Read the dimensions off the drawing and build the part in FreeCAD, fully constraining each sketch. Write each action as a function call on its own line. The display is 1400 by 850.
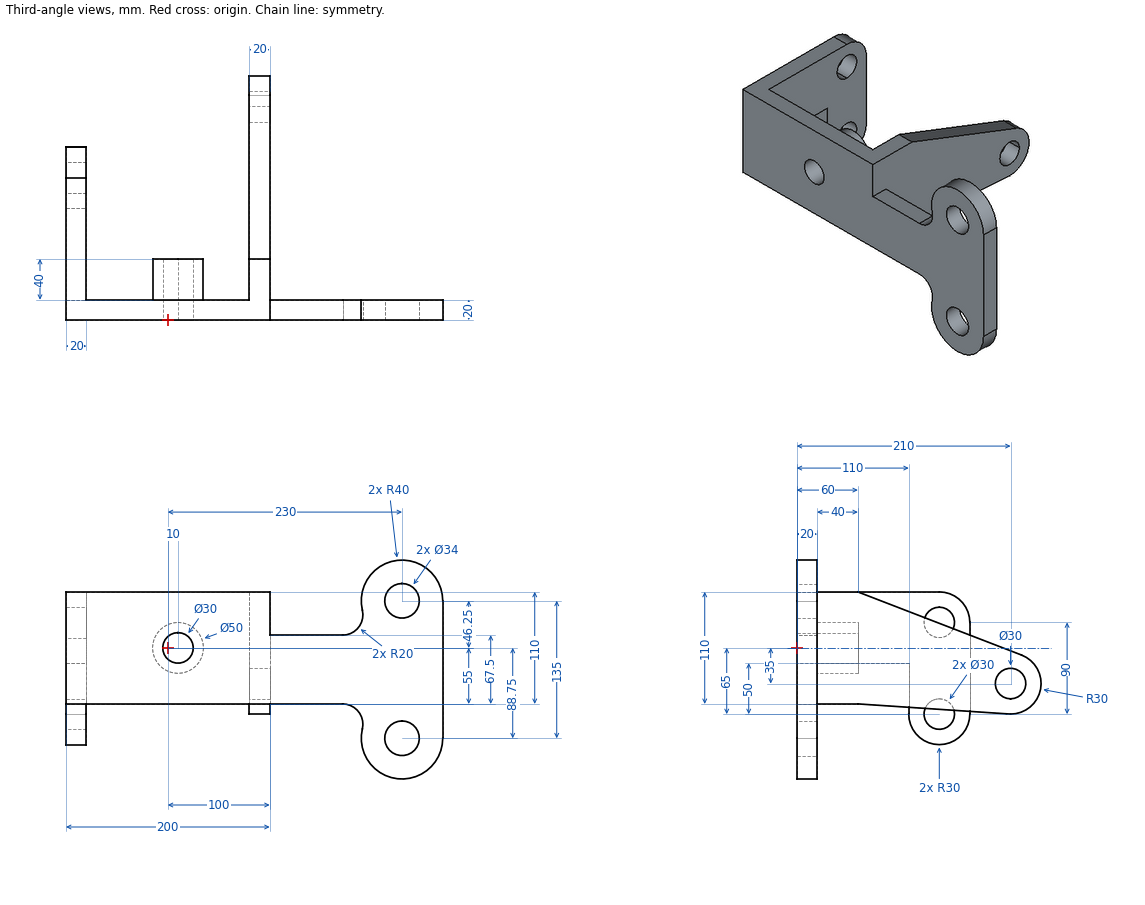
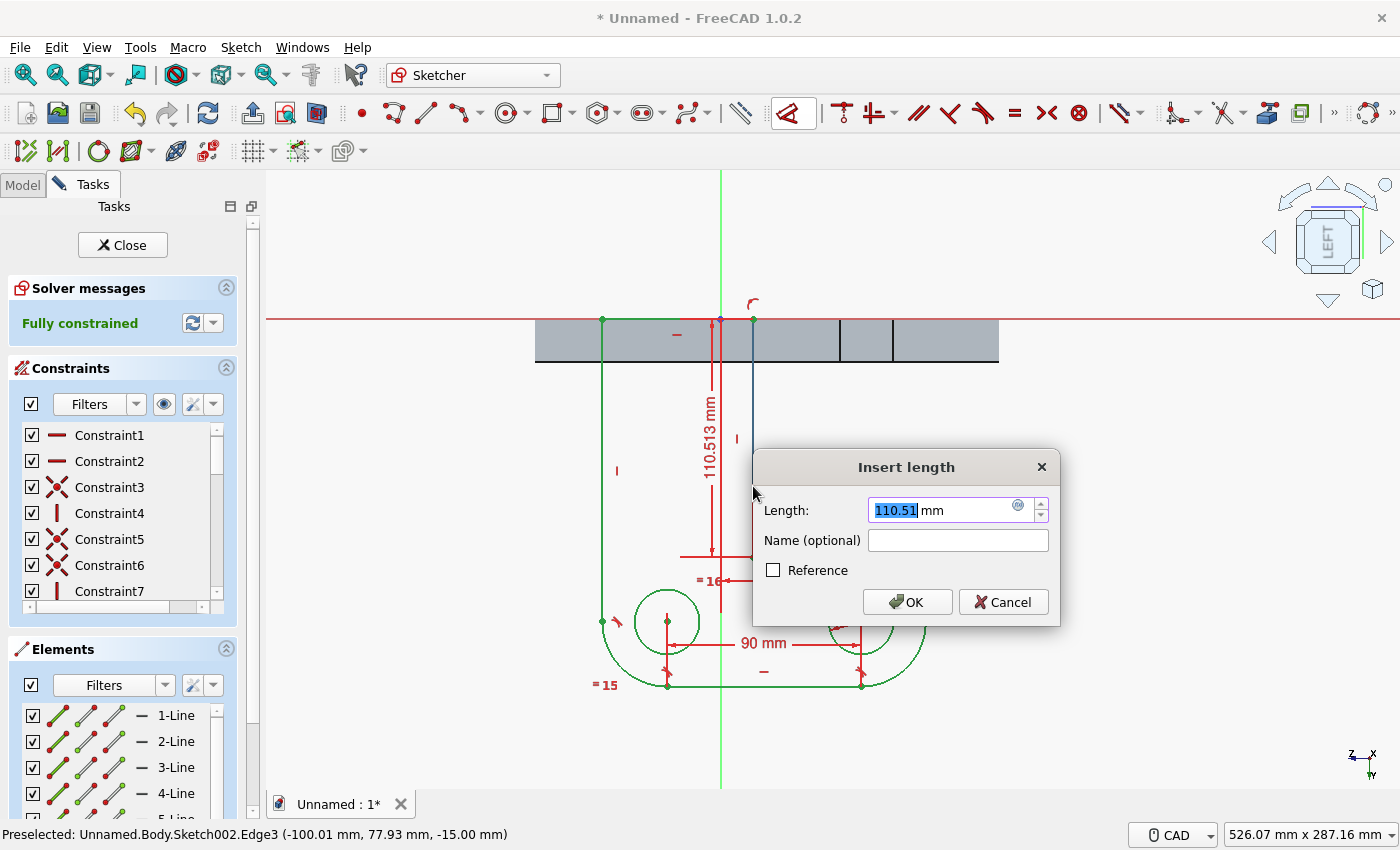
text(110)
key(Return)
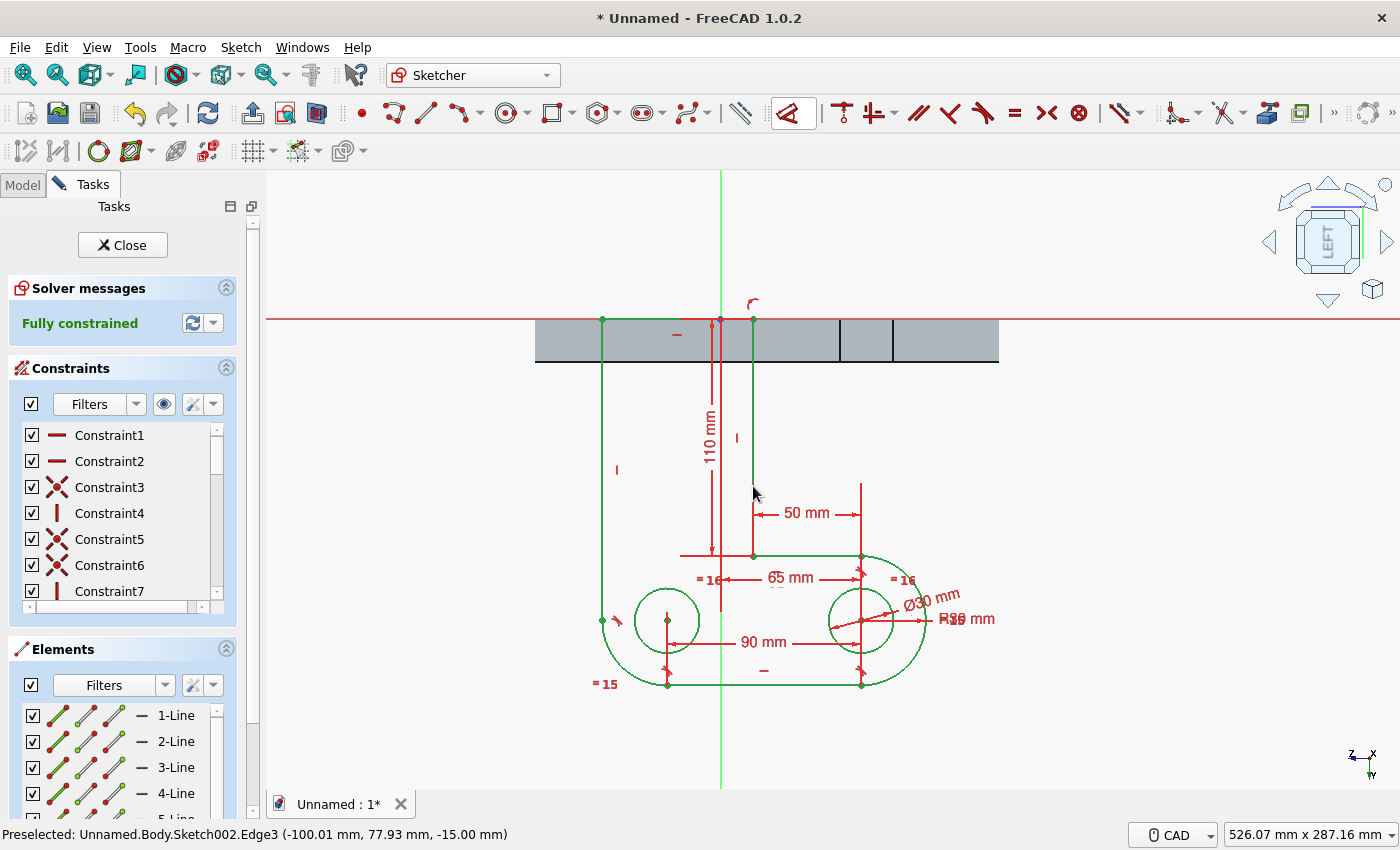
click(123, 245)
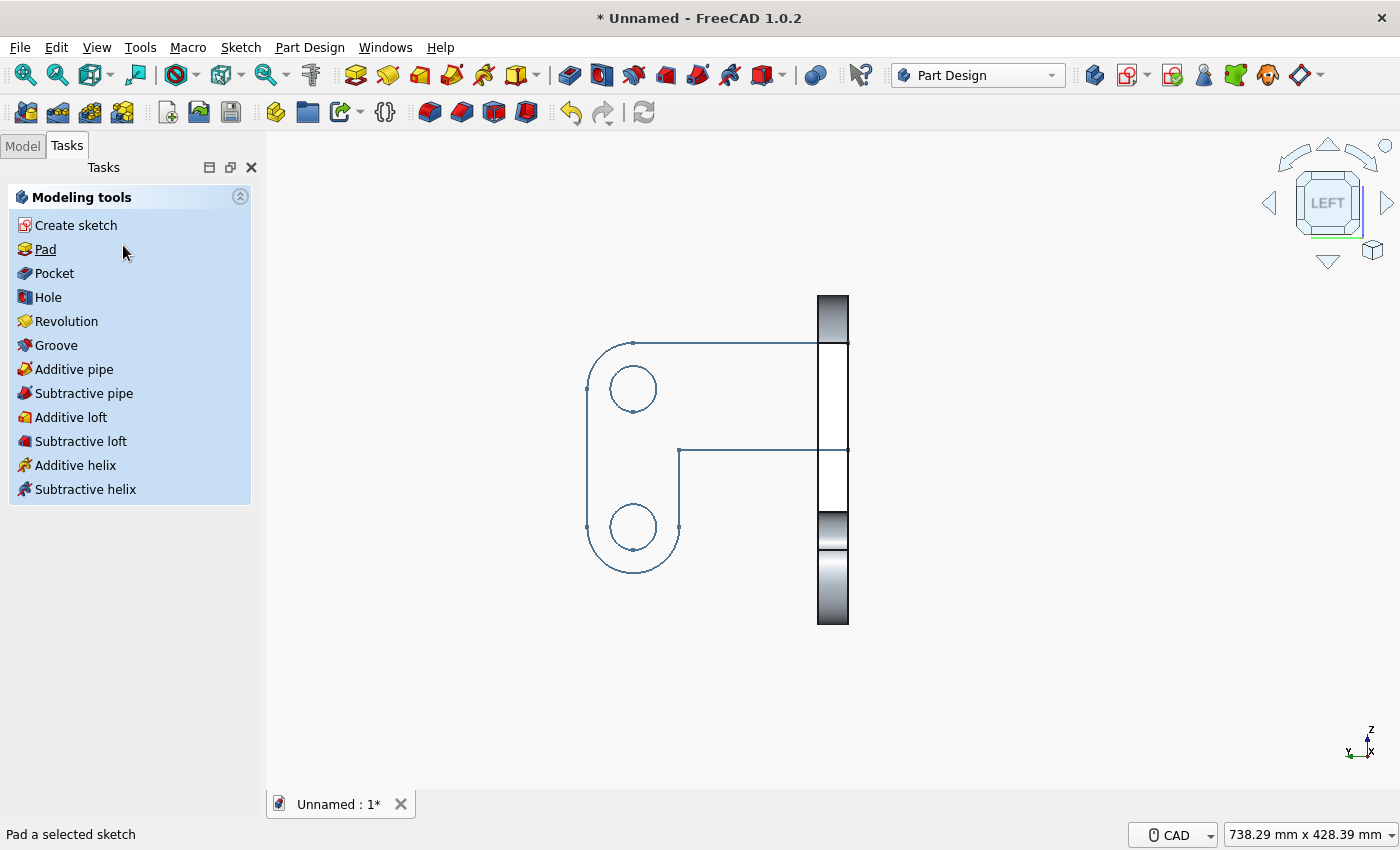
click(356, 76)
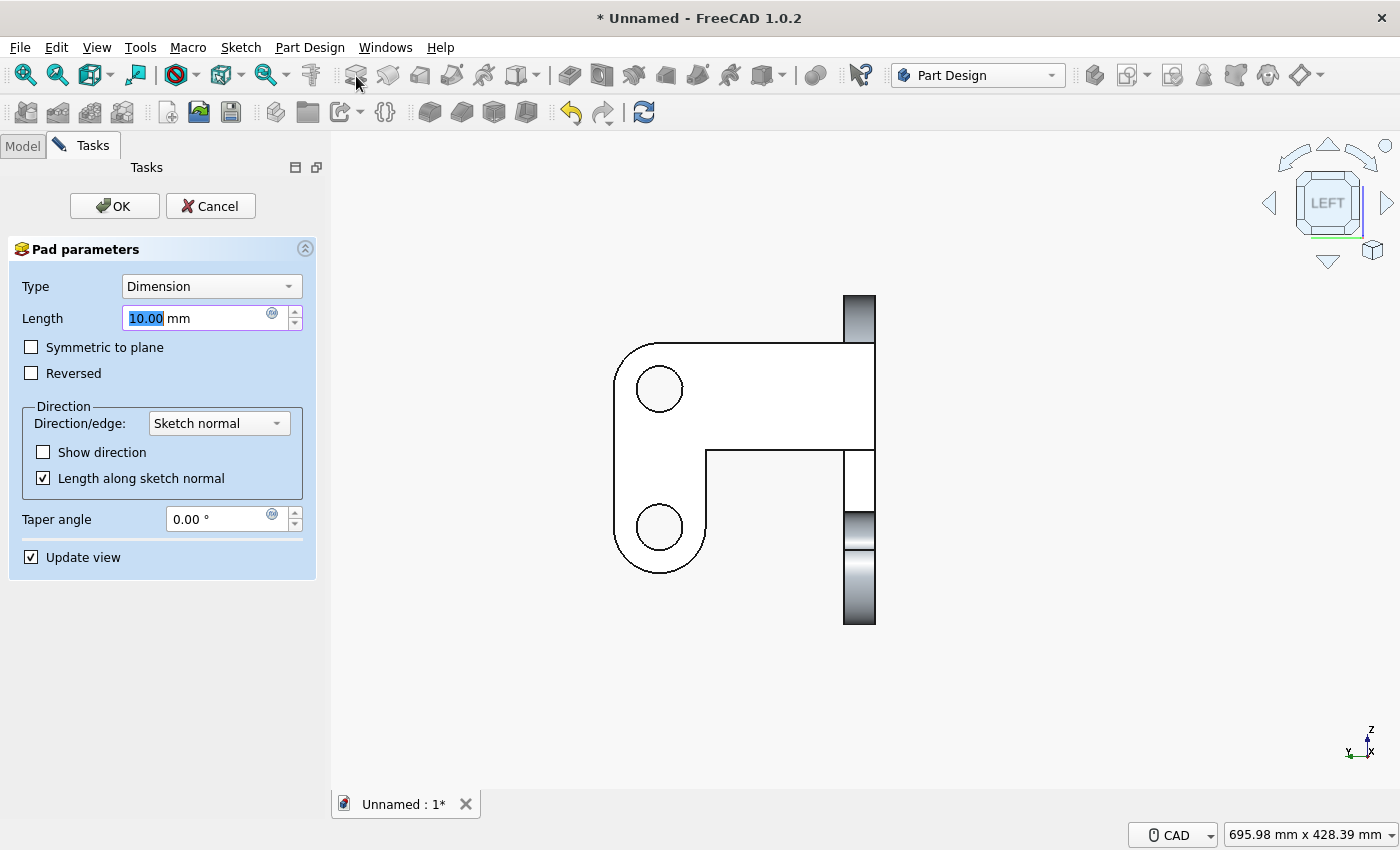
text(20)
key(Tab)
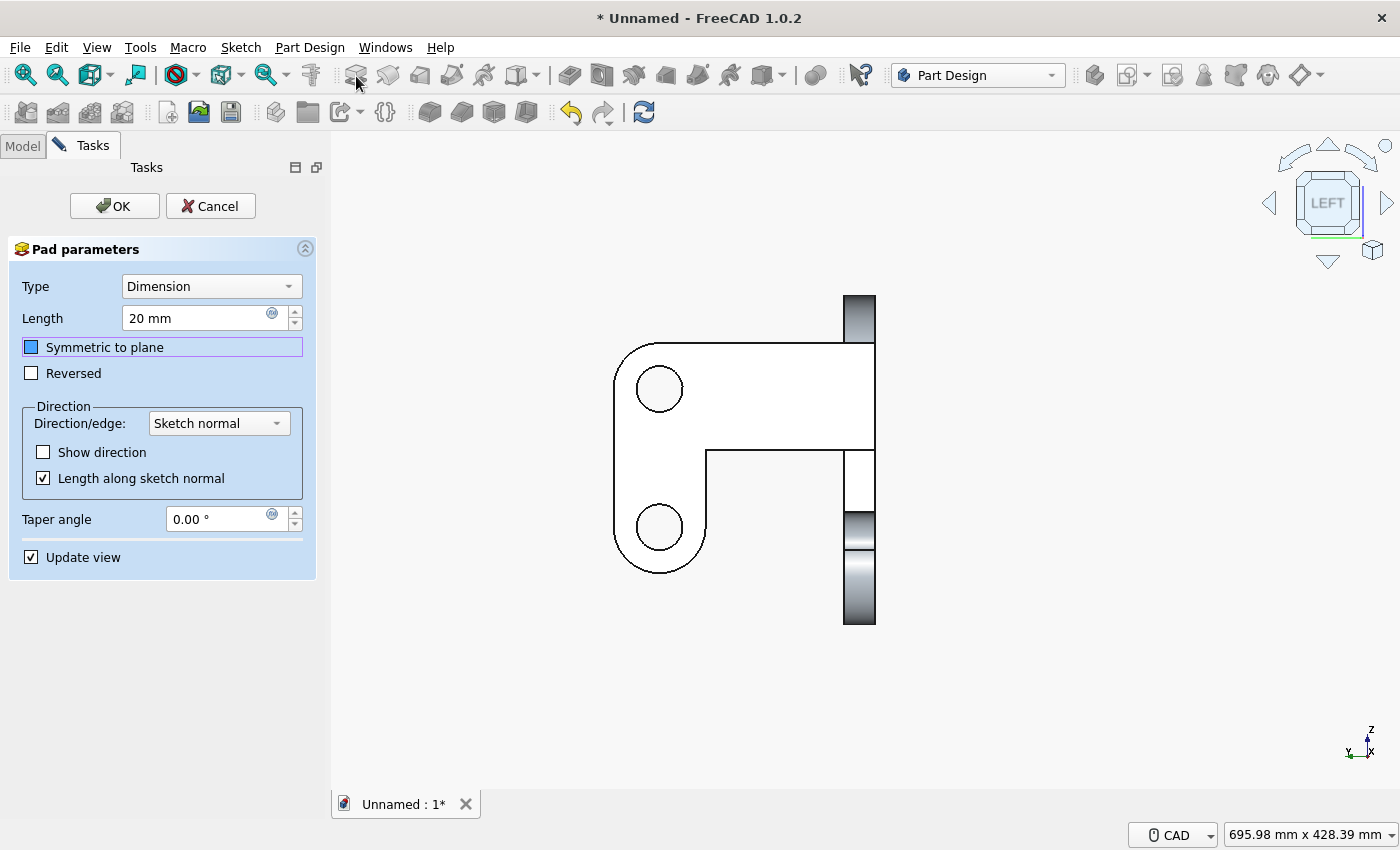
click(30, 373)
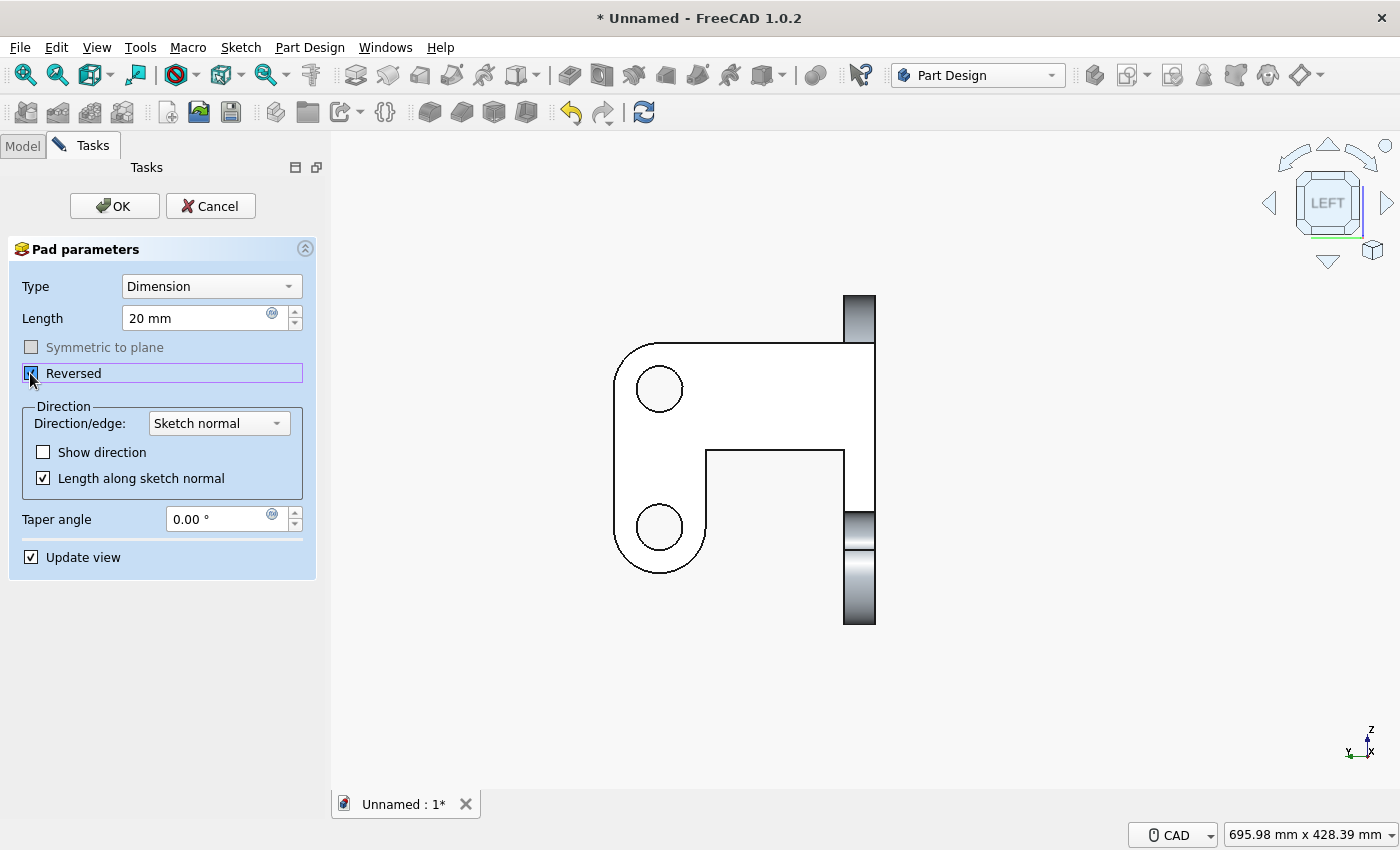
click(115, 206)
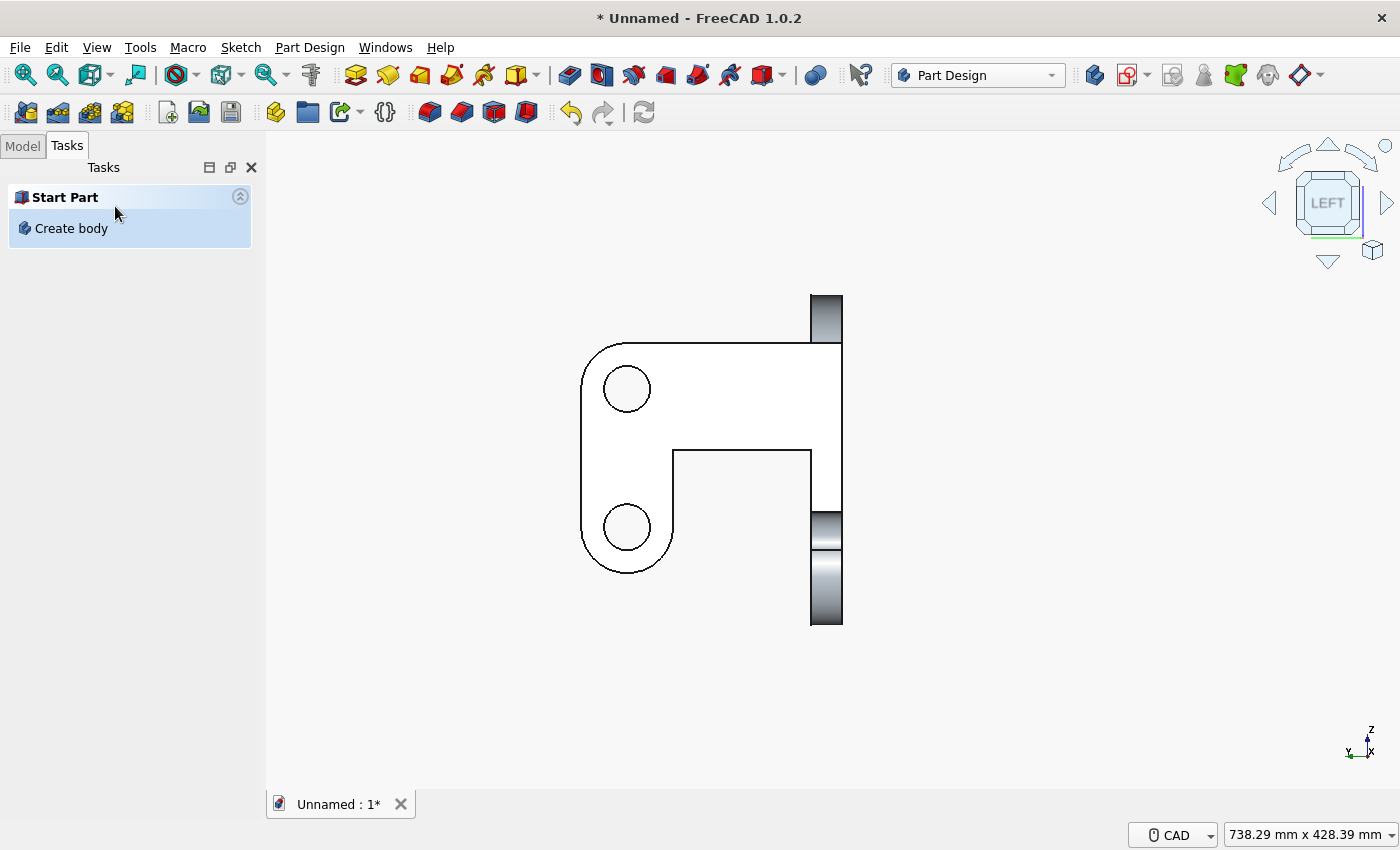
click(23, 145)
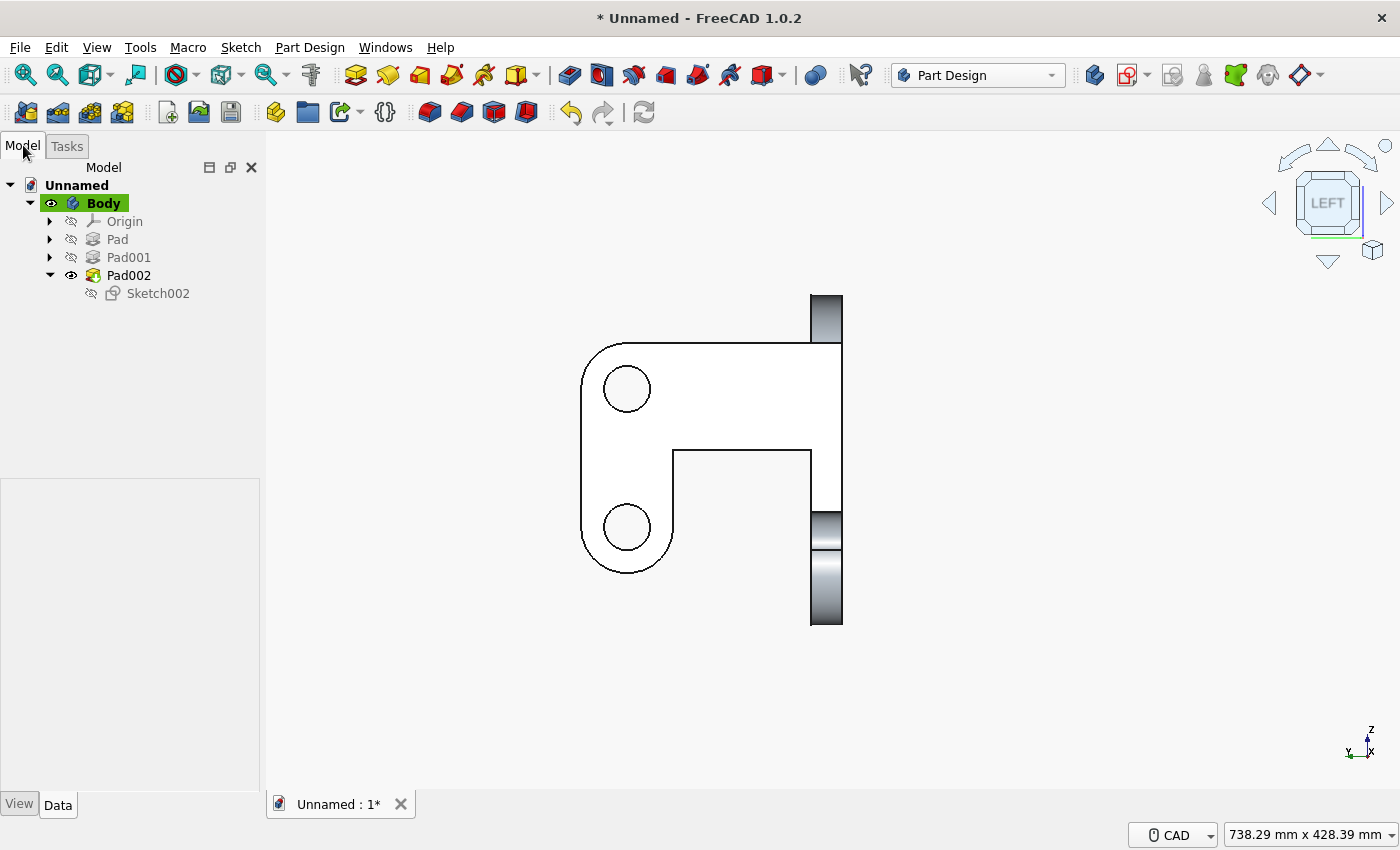
click(50, 221)